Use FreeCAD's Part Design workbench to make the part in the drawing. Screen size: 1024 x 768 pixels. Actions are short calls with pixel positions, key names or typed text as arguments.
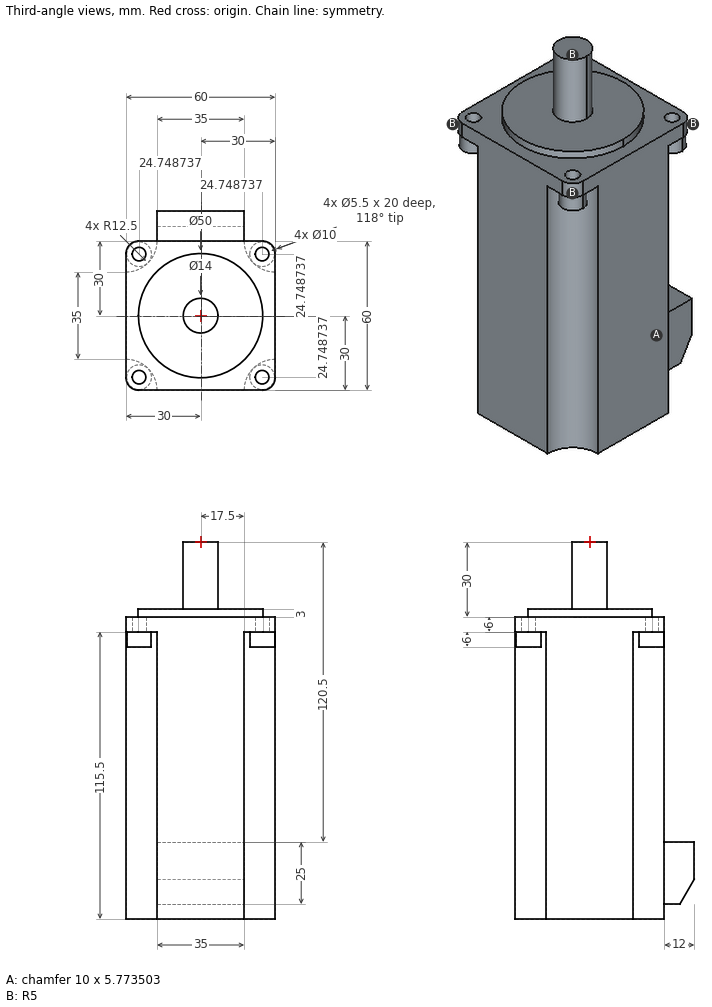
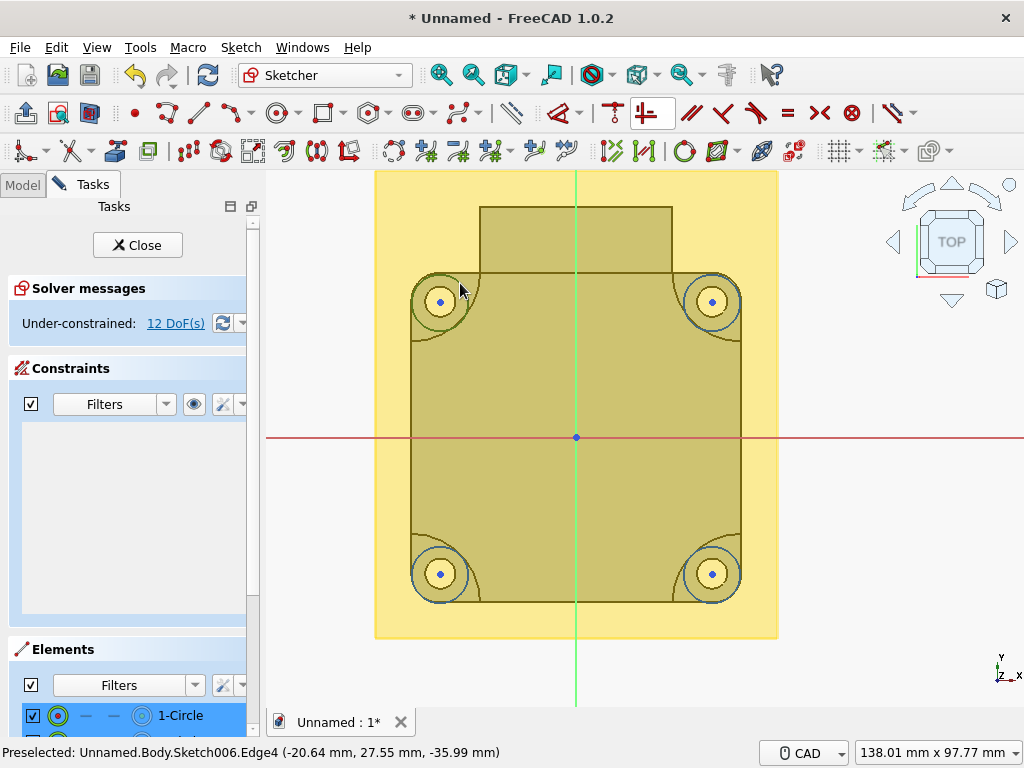
click(788, 114)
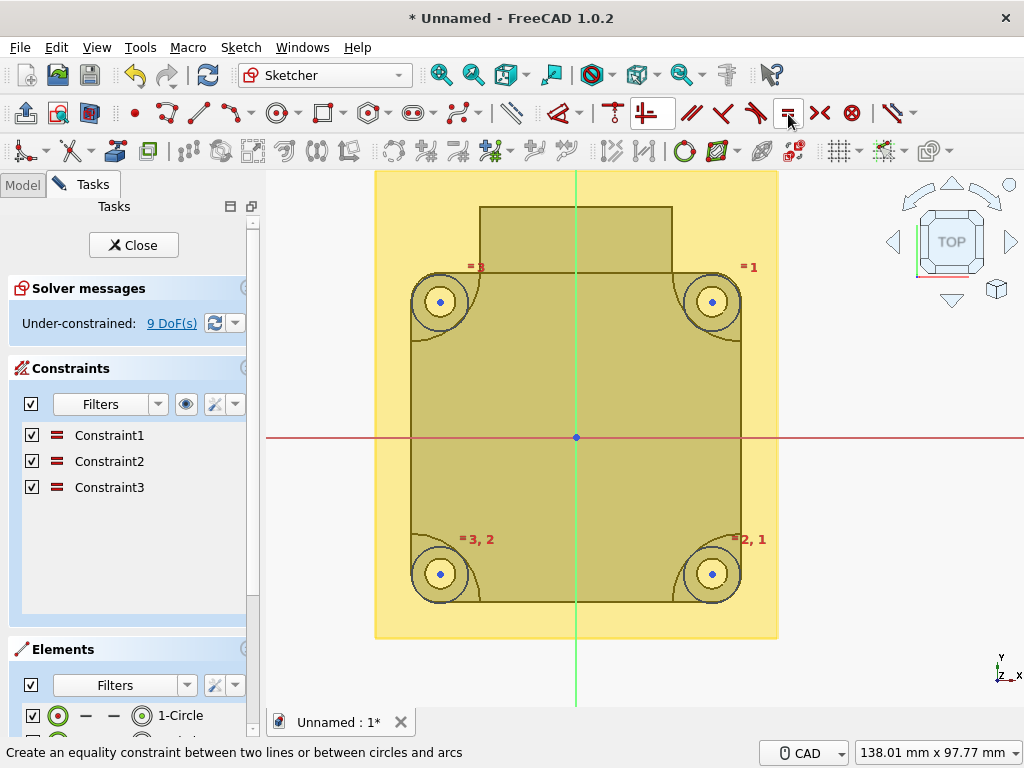
click(712, 303)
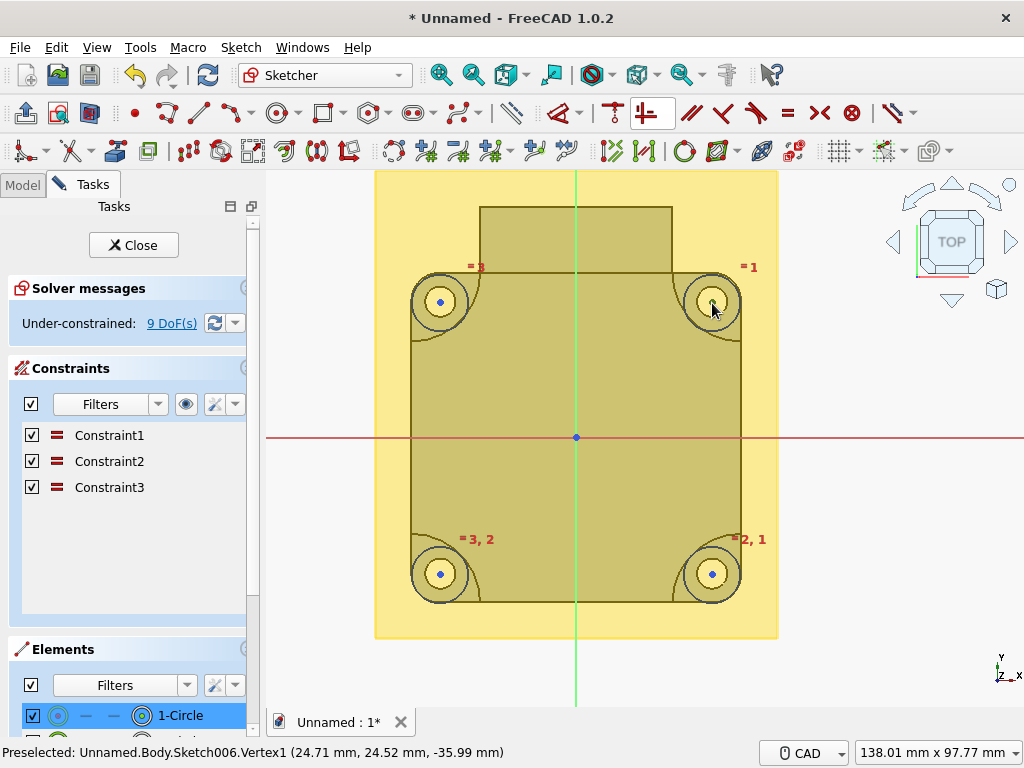
click(712, 575)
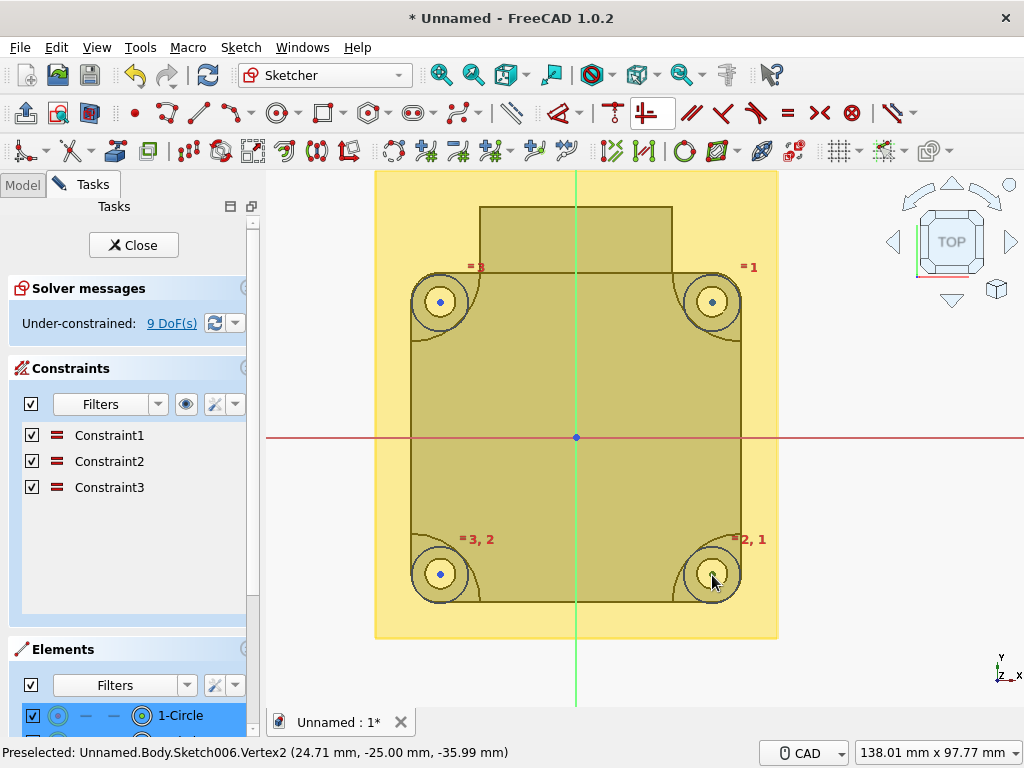
key(v)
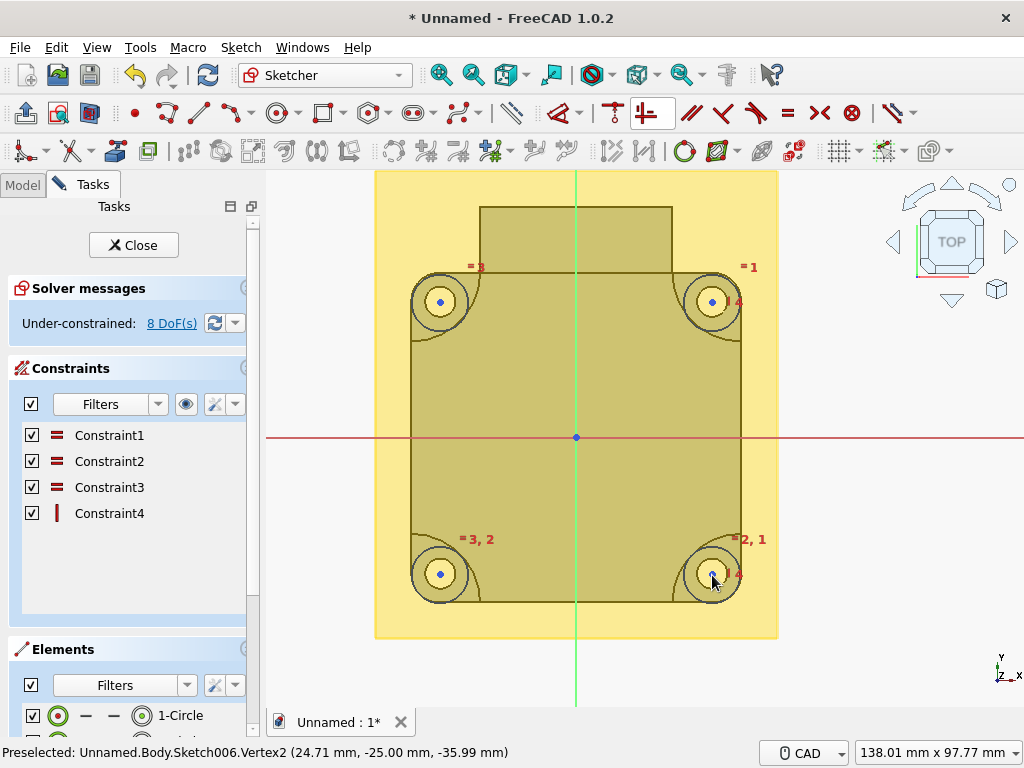
click(712, 575)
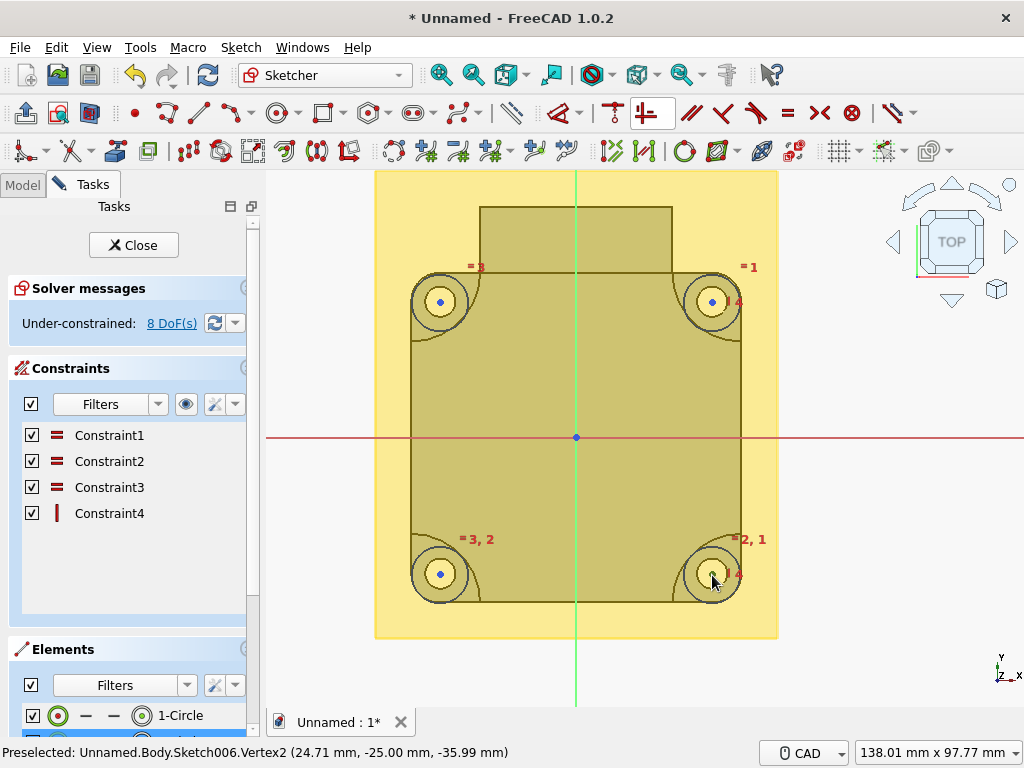
click(440, 575)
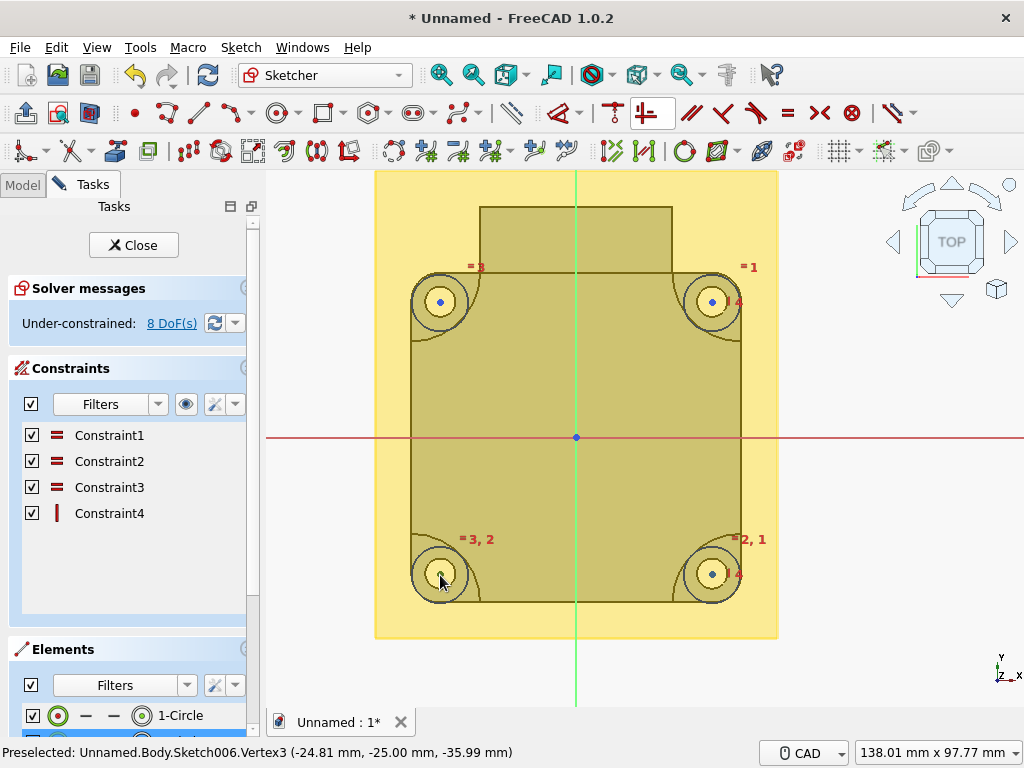
click(670, 114)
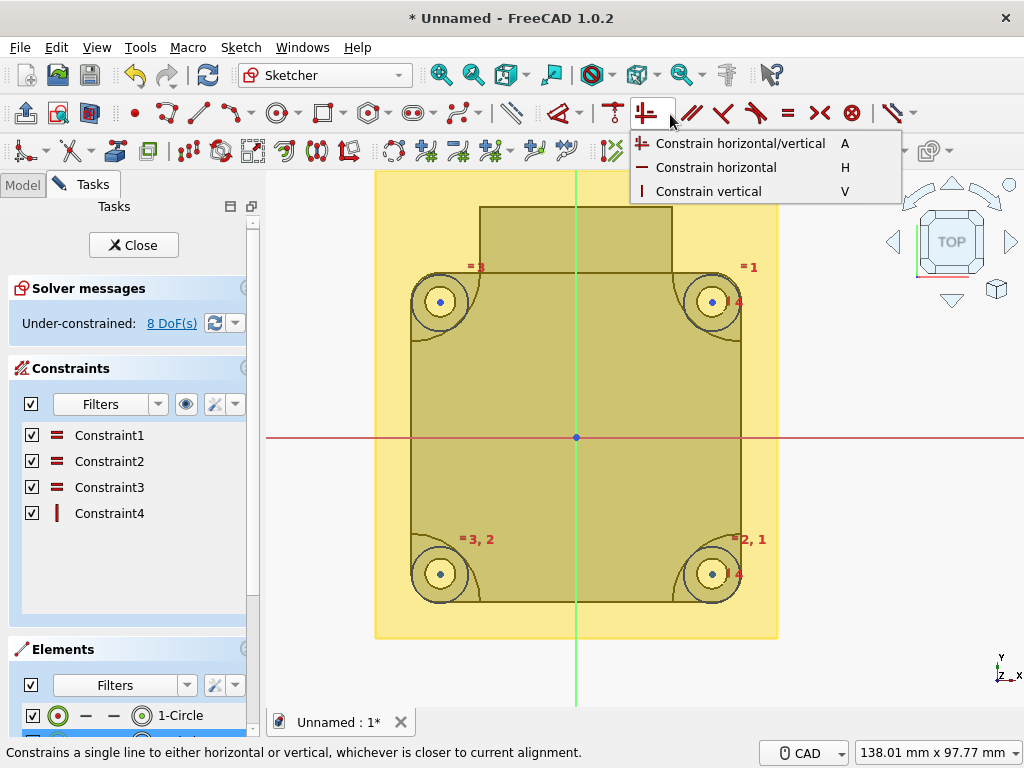
click(766, 167)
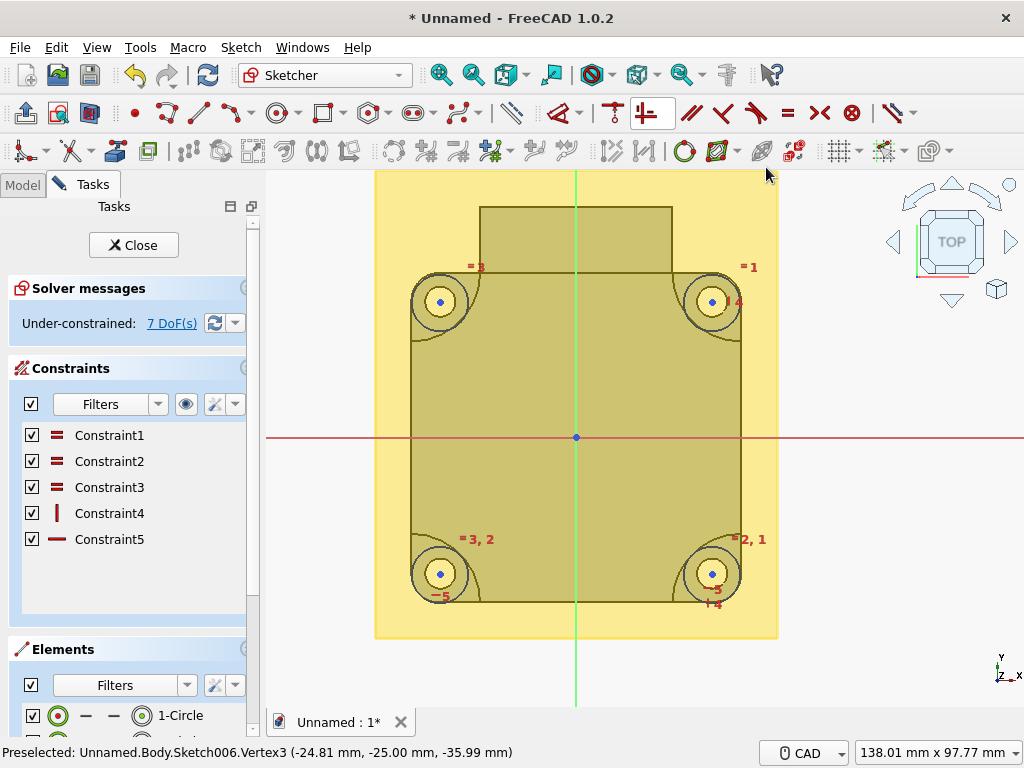
click(440, 575)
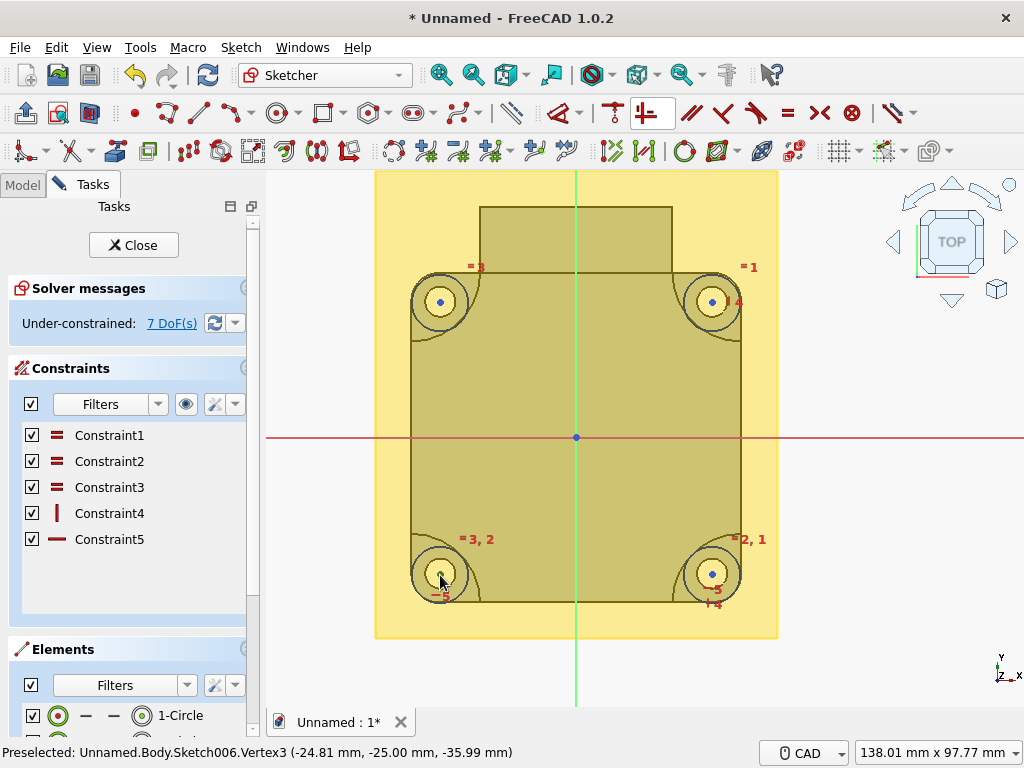
click(440, 303)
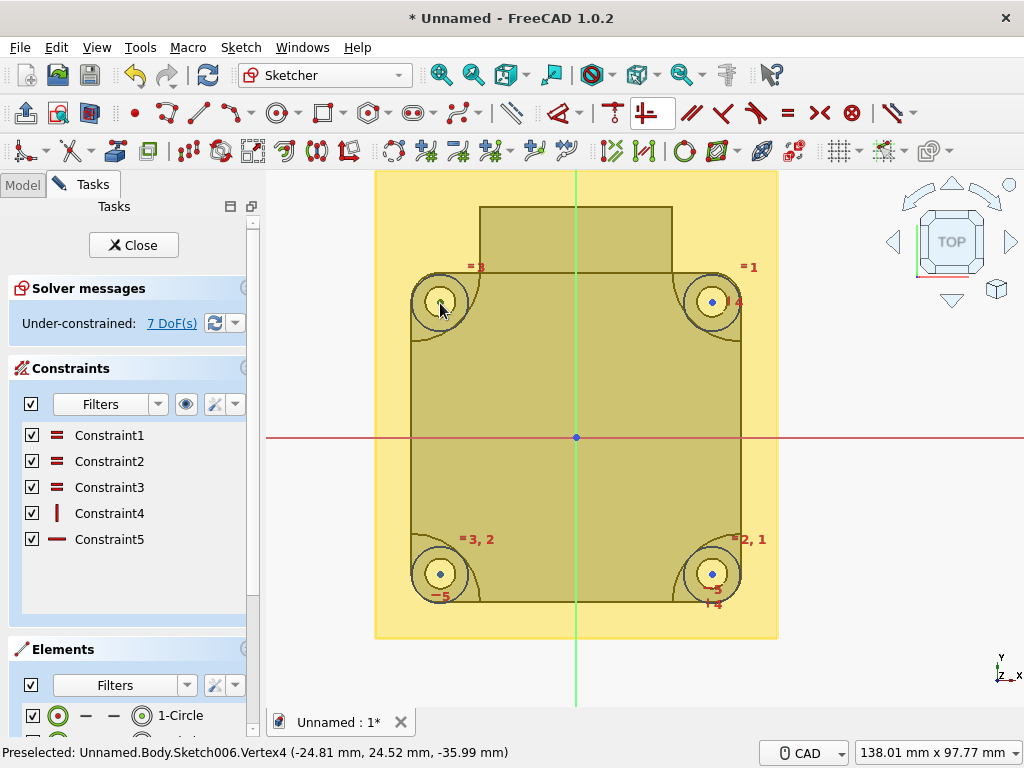
click(670, 114)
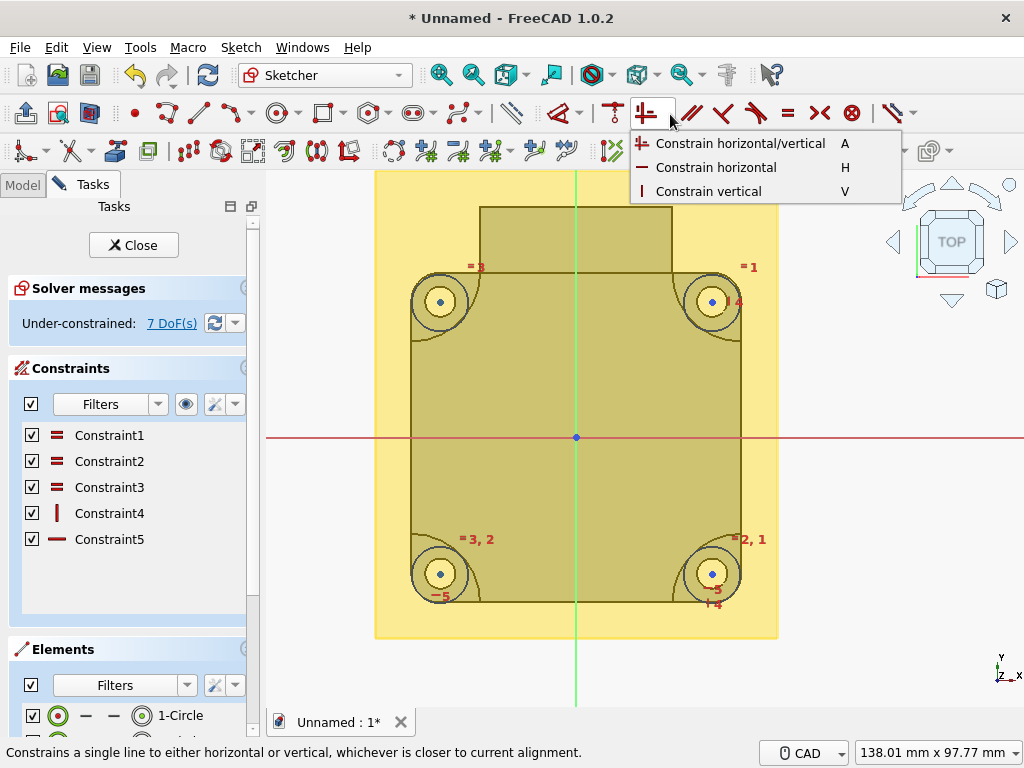
click(766, 191)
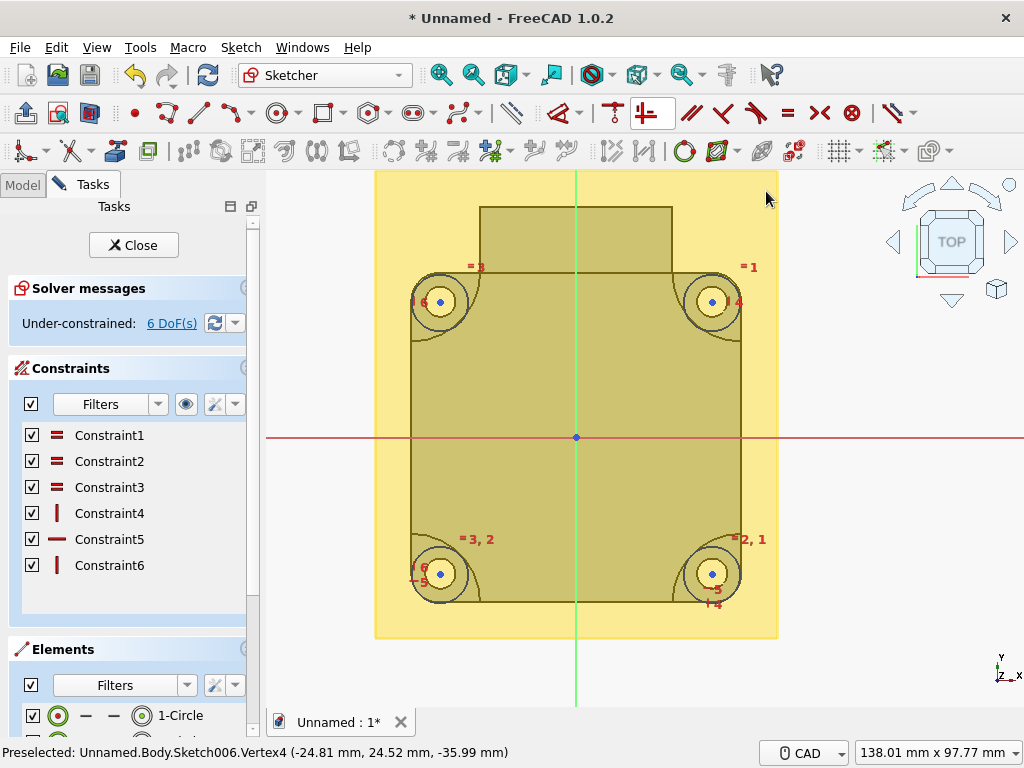
click(712, 303)